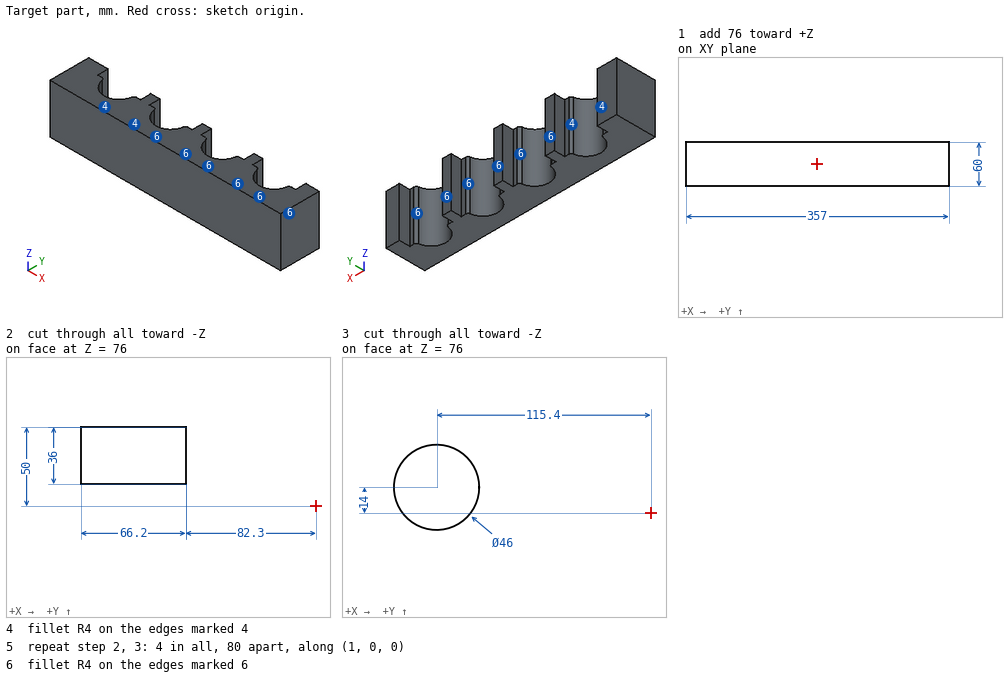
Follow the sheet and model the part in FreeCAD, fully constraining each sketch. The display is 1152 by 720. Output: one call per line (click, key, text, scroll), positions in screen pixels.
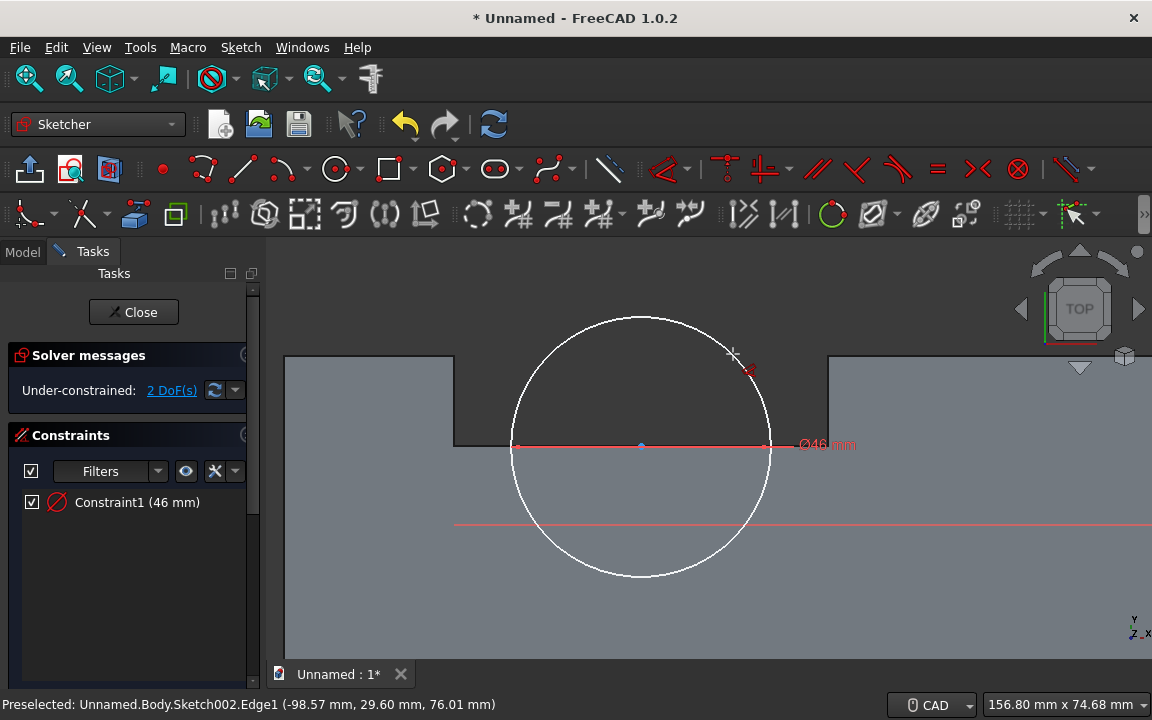
click(641, 447)
click(607, 486)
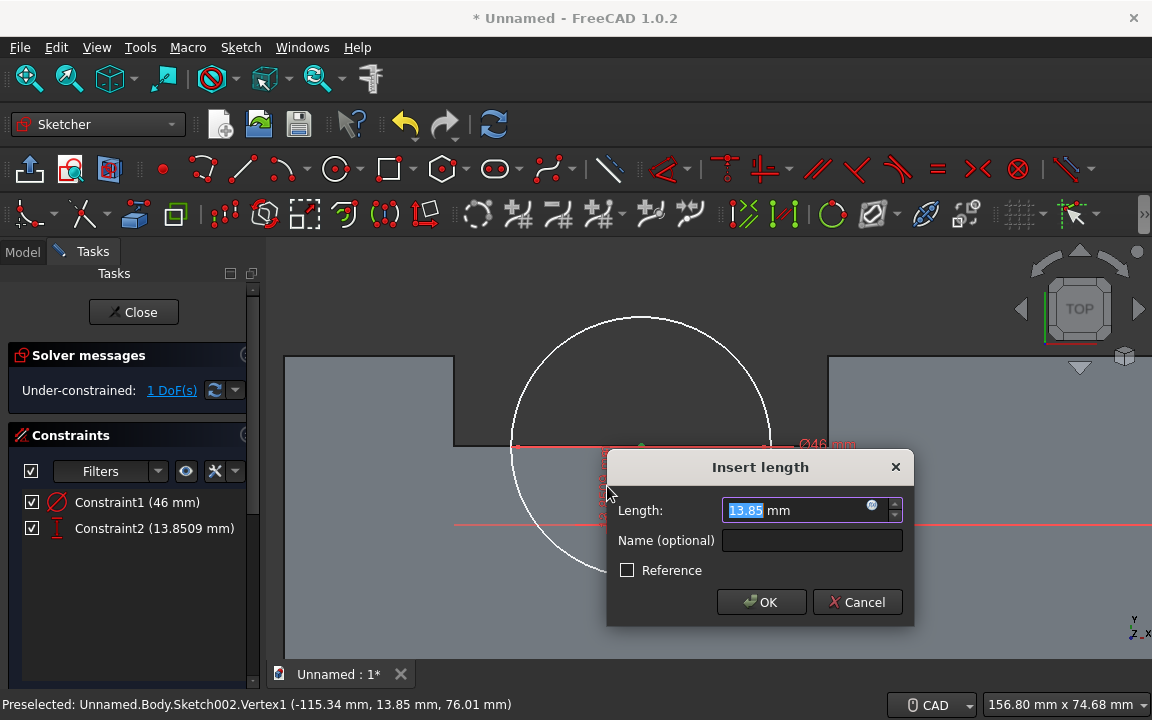
text(14)
key(Return)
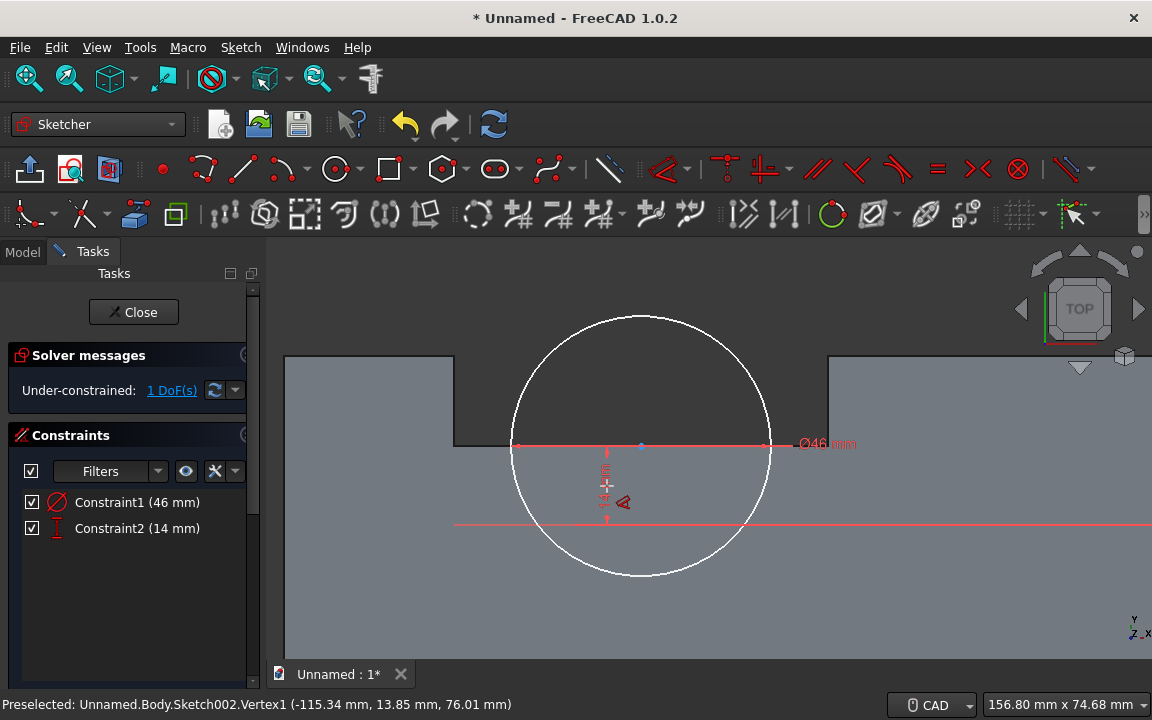
click(641, 446)
click(814, 559)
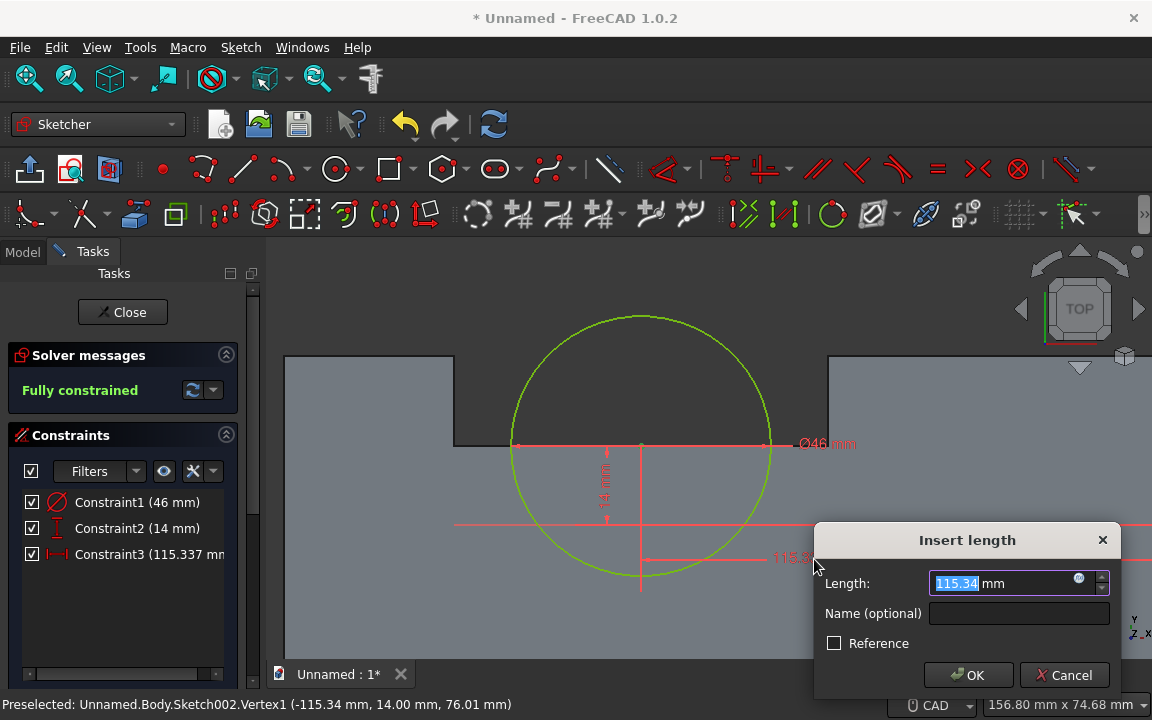
text(115.4)
key(Return)
key(Escape)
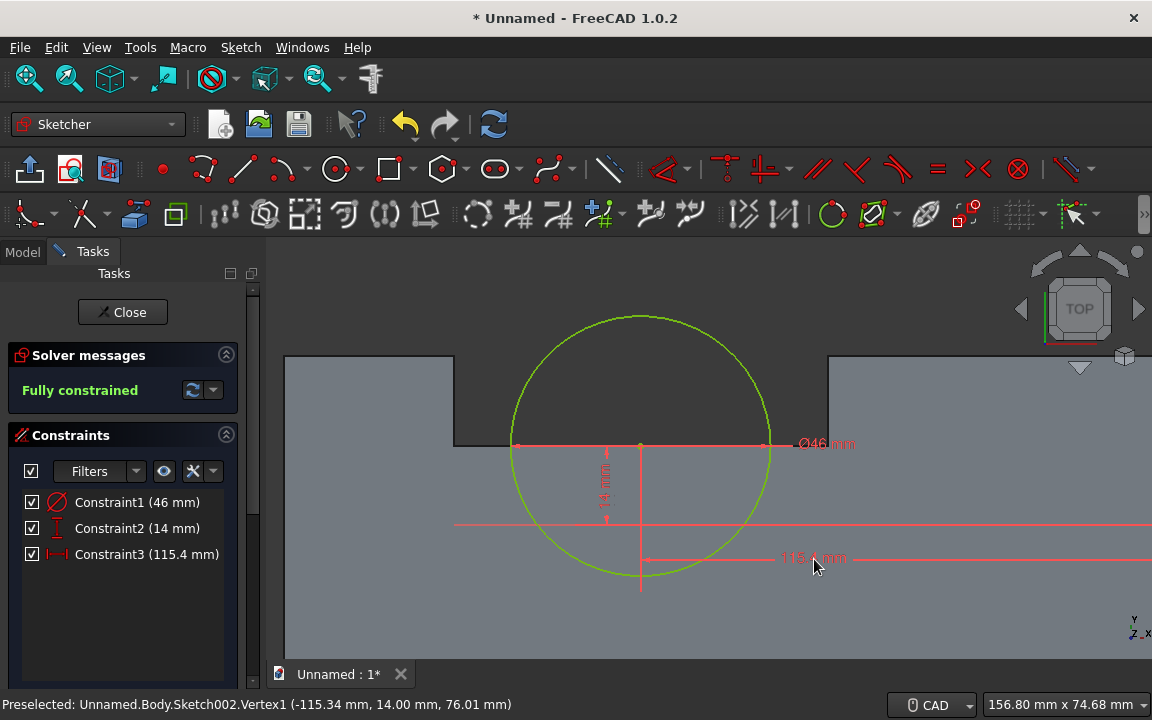
click(123, 312)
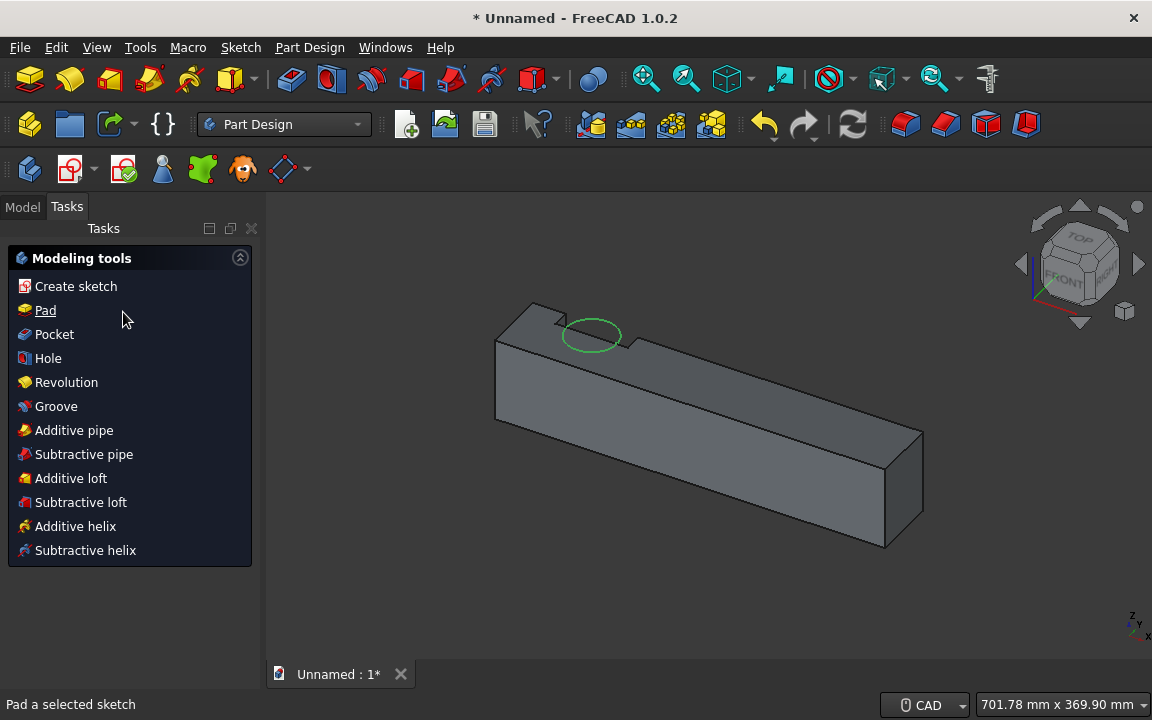
click(292, 80)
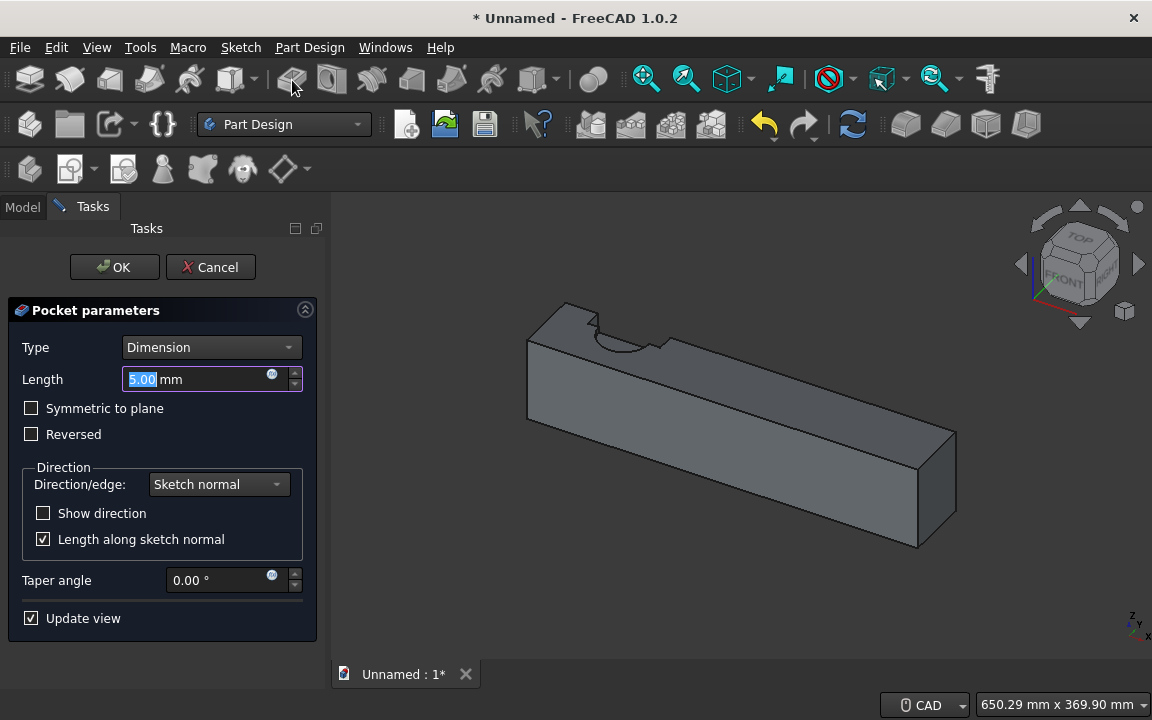
click(212, 348)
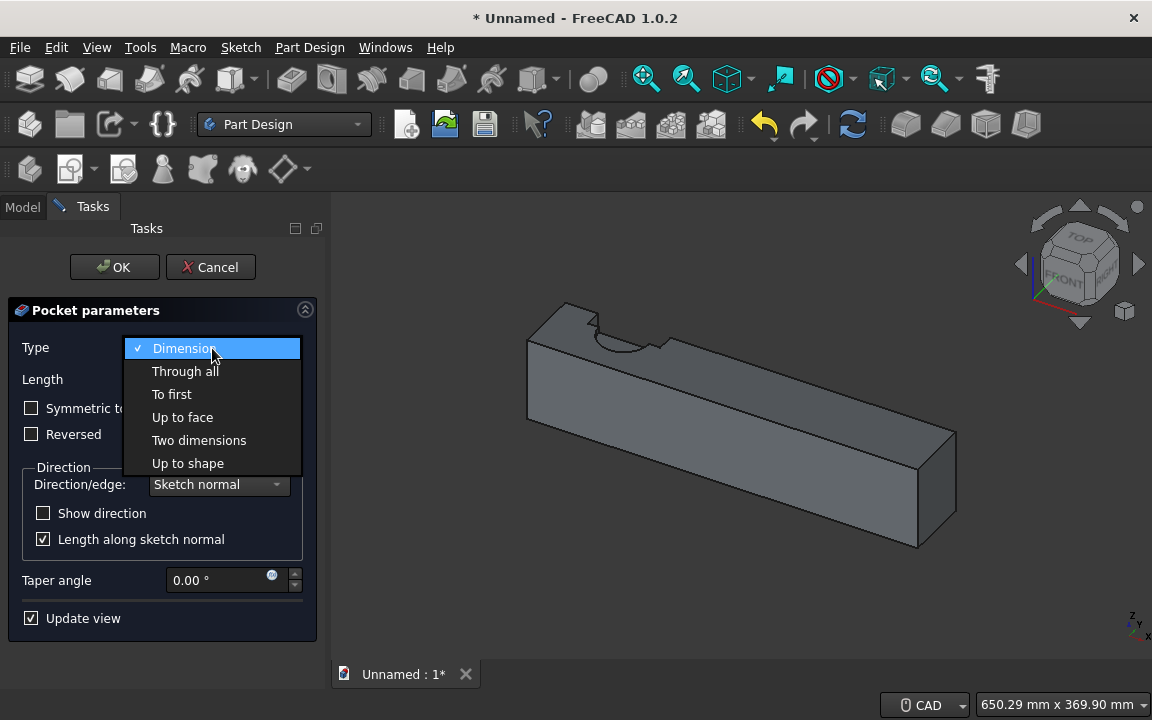
click(212, 372)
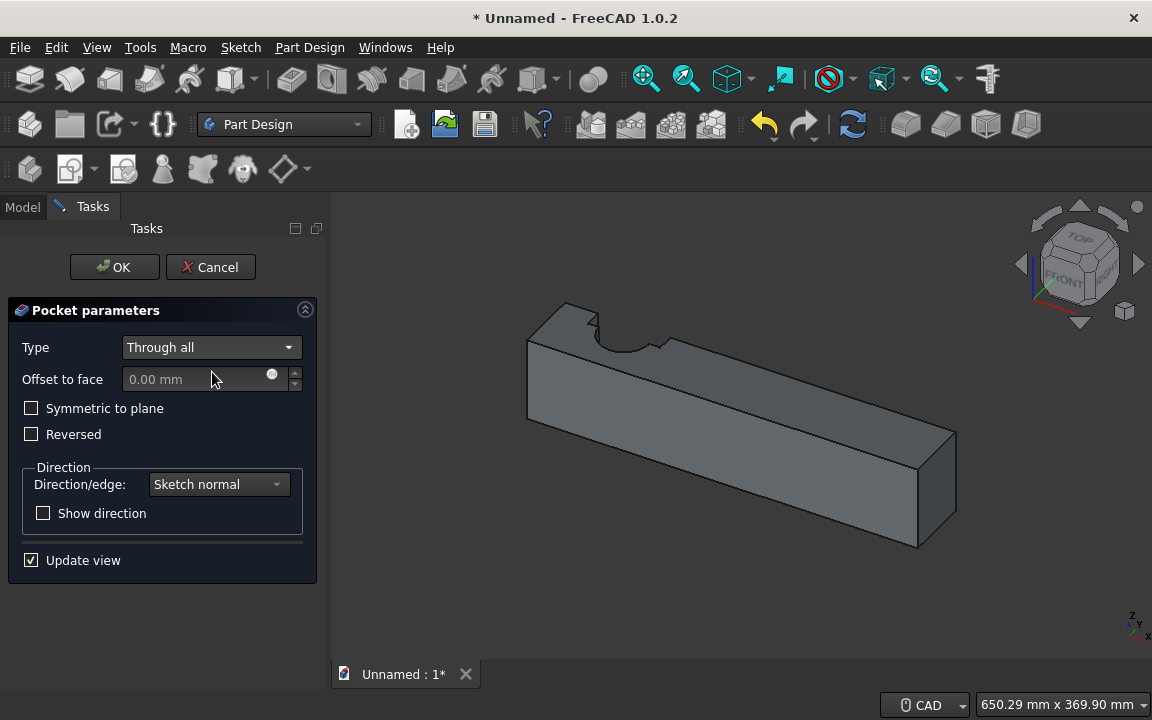
click(115, 267)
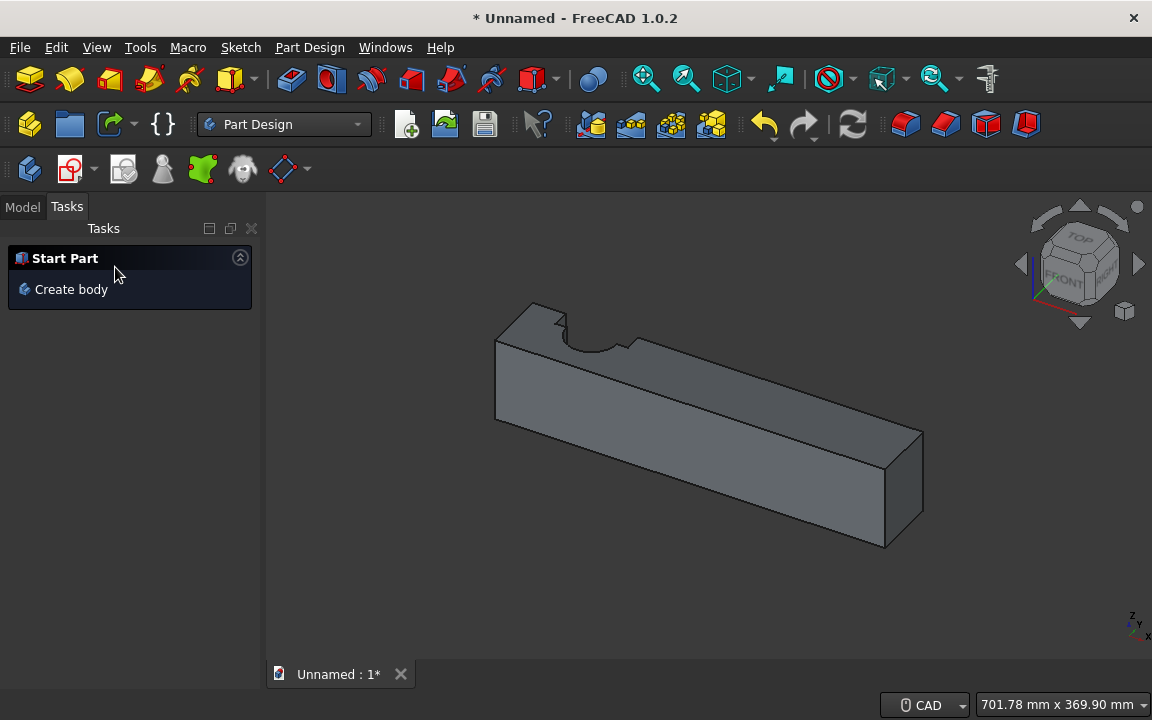
key(0)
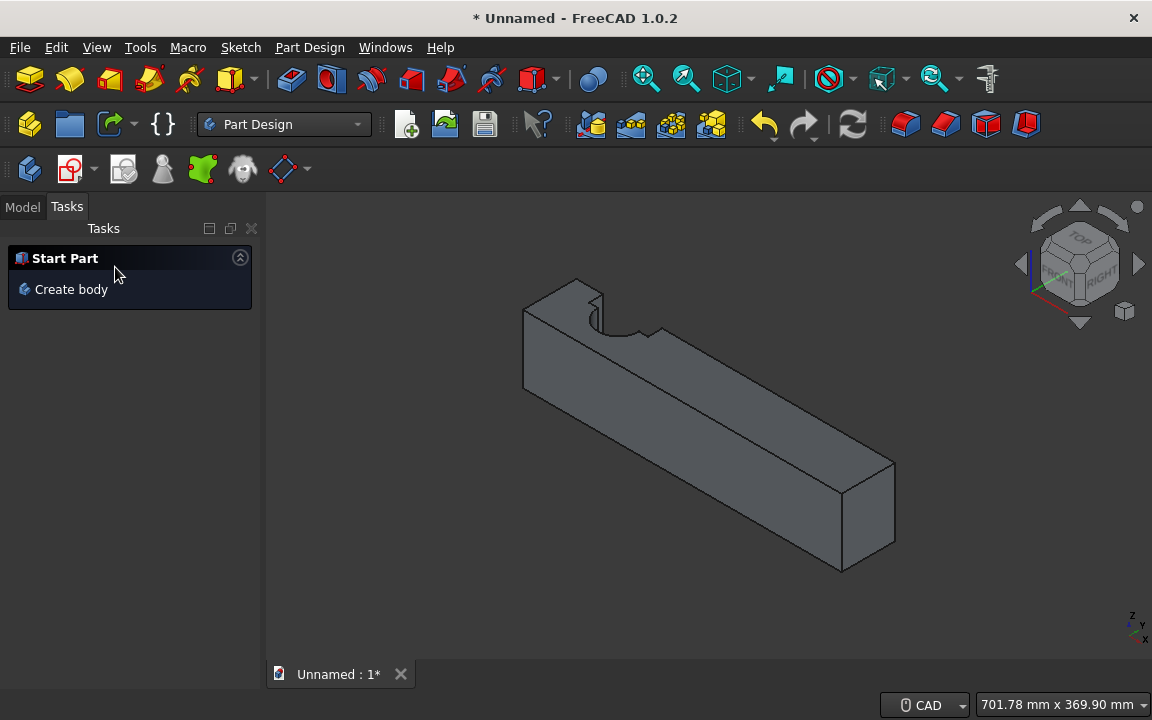
key(2)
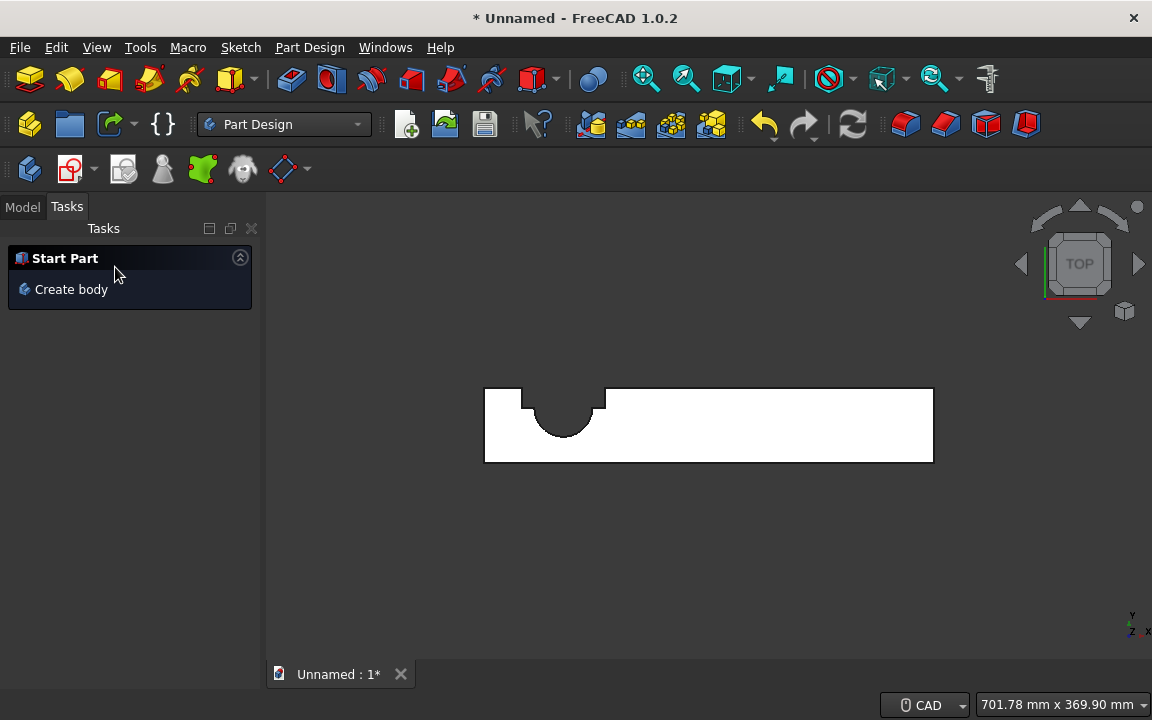
key(1)